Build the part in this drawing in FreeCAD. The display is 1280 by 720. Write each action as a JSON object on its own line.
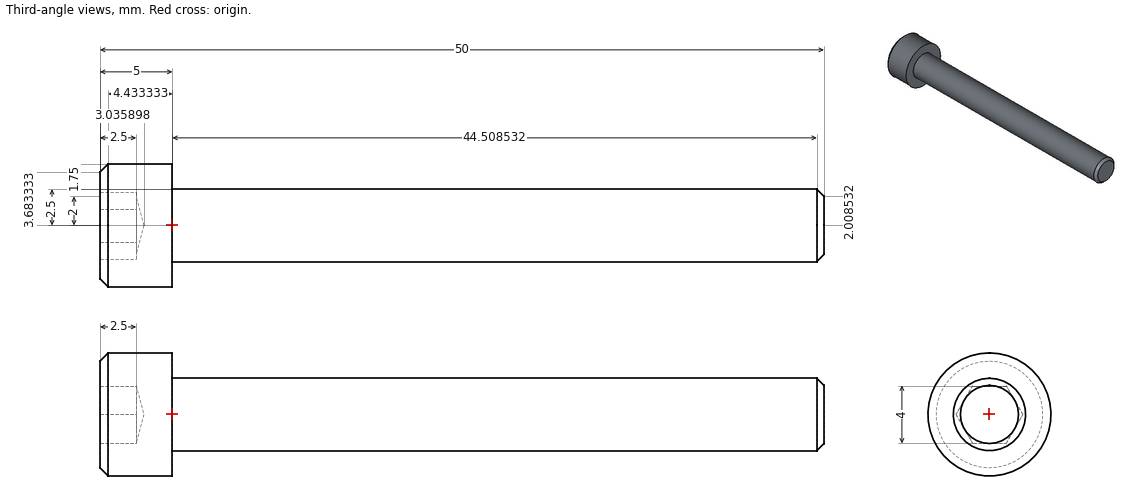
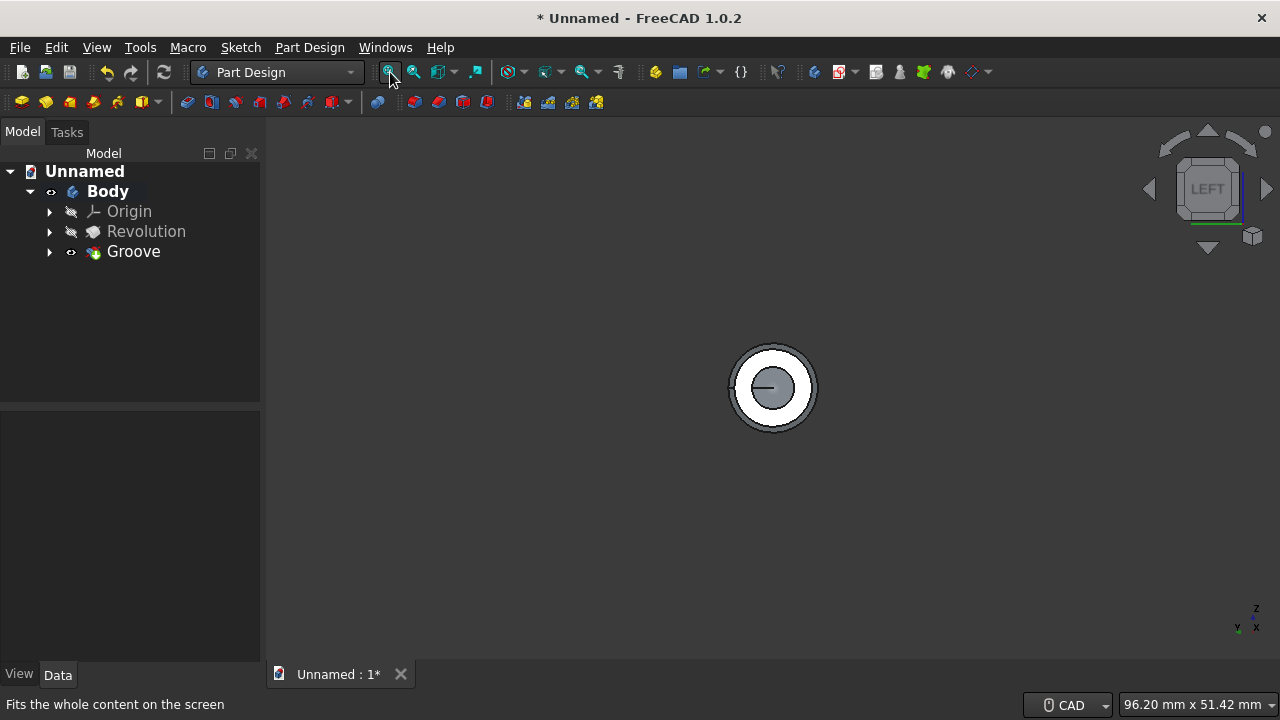
{"action": "key", "text": "2"}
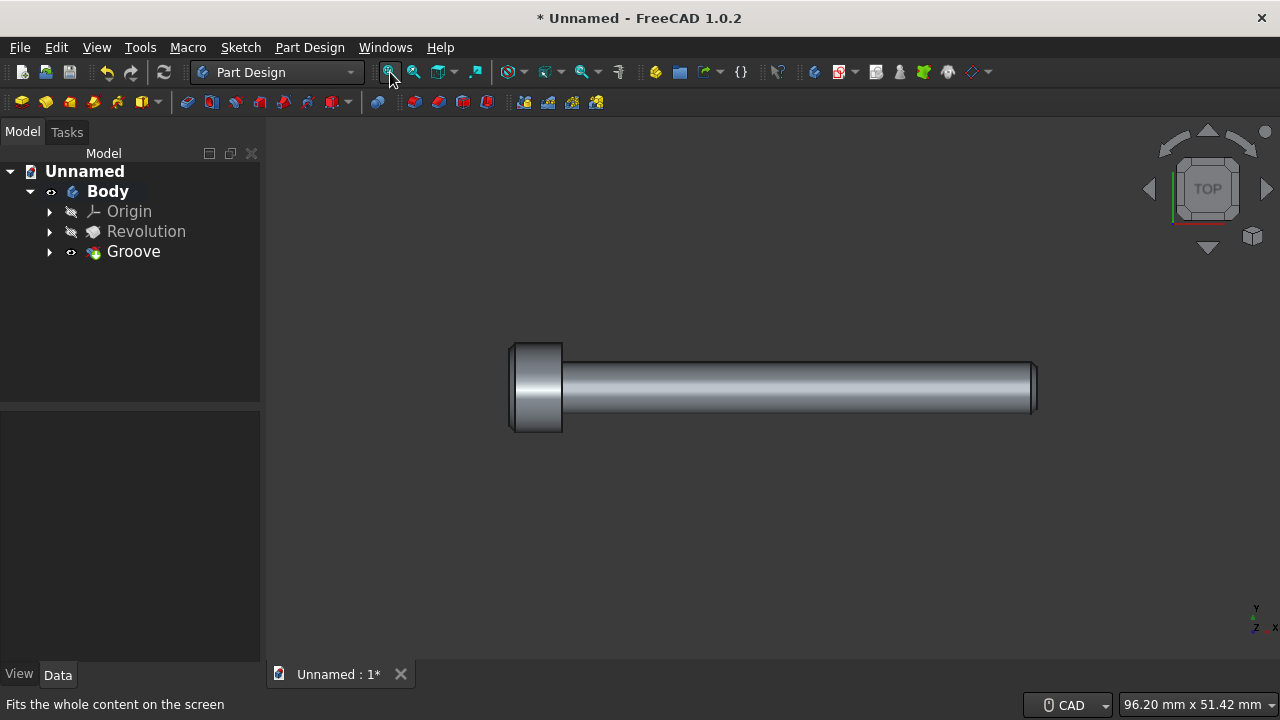
{"action": "key", "text": "1"}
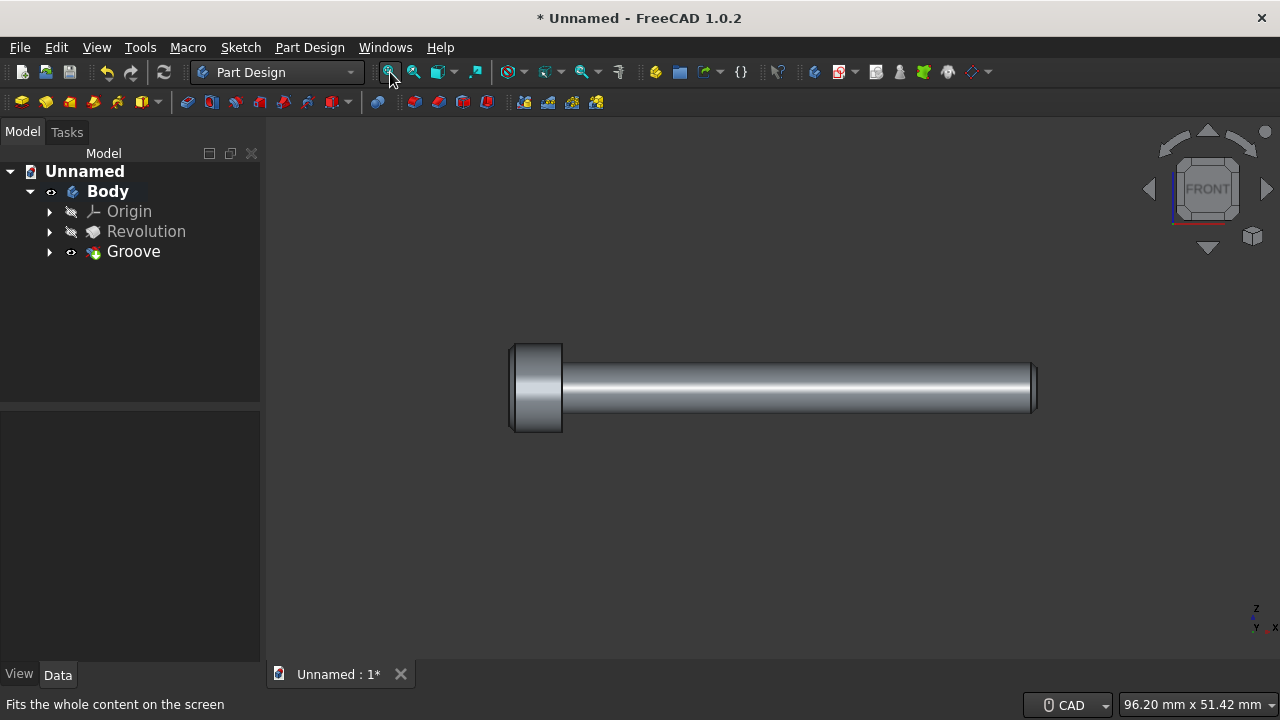
{"action": "left_click", "coordinate": [50, 212]}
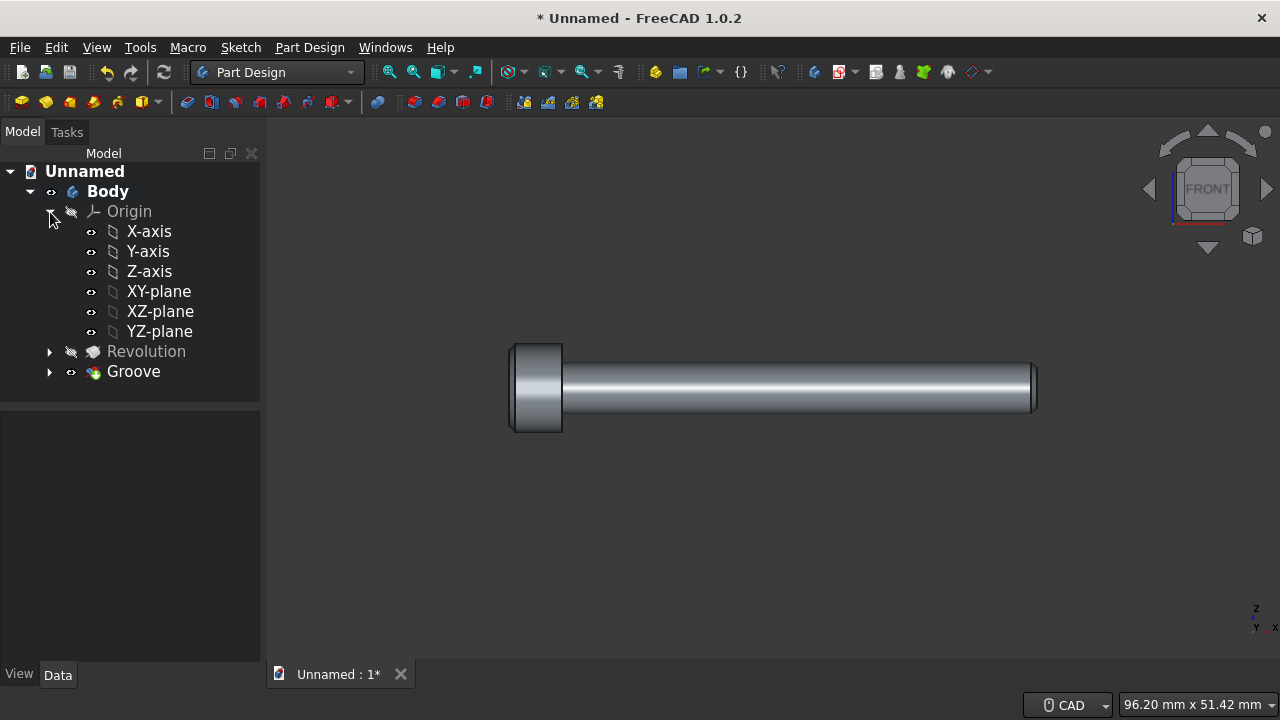
{"action": "left_click", "coordinate": [136, 332]}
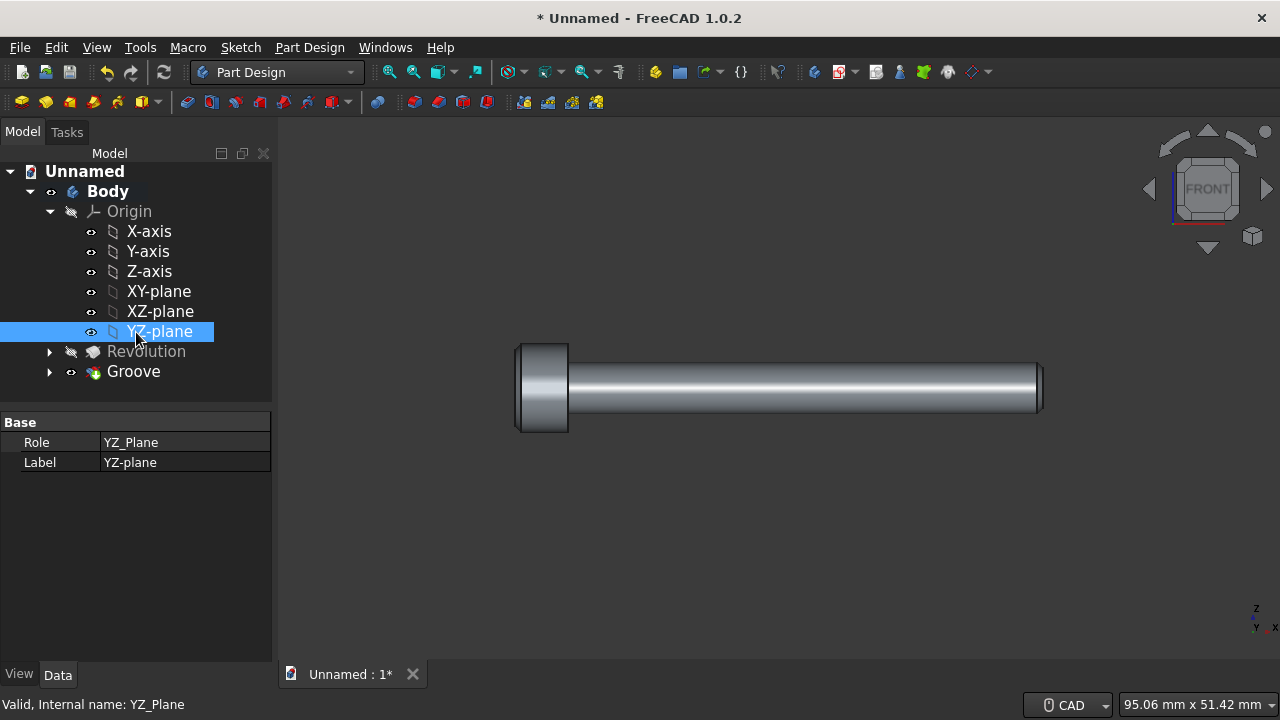
{"action": "left_click", "coordinate": [972, 72]}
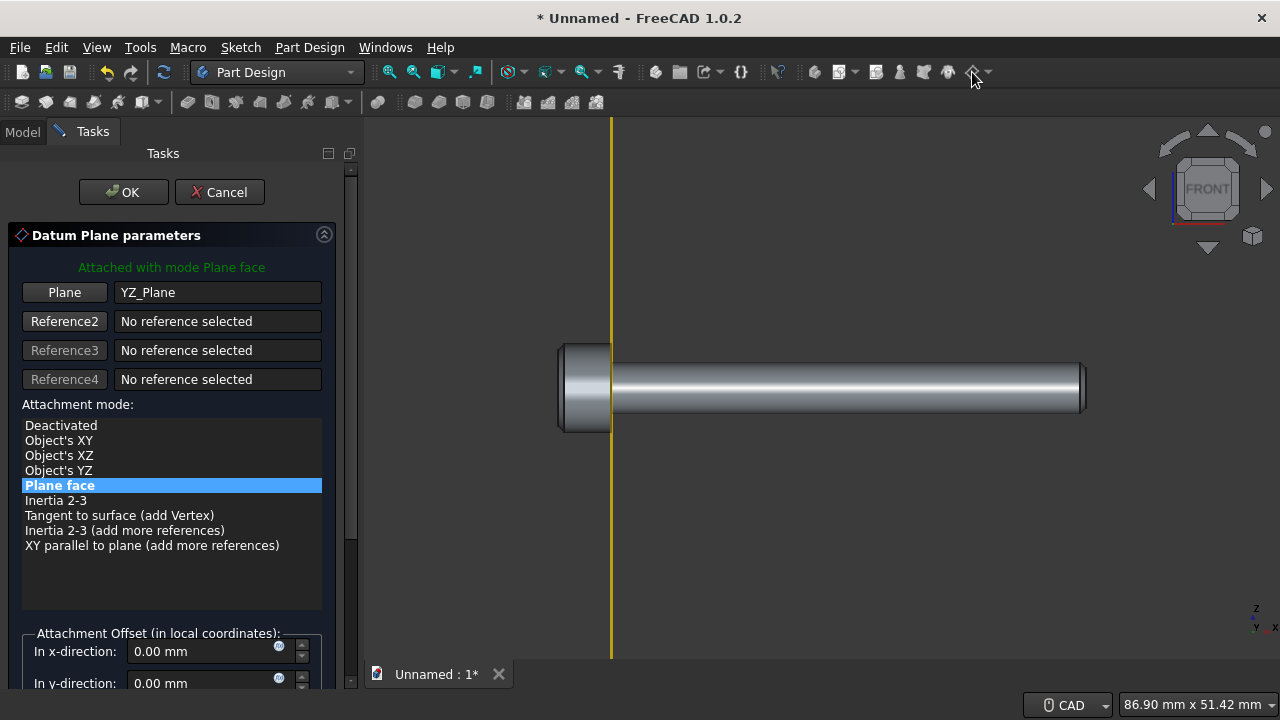
{"action": "scroll", "coordinate": [351, 426], "scroll_direction": "down", "scroll_amount": 2}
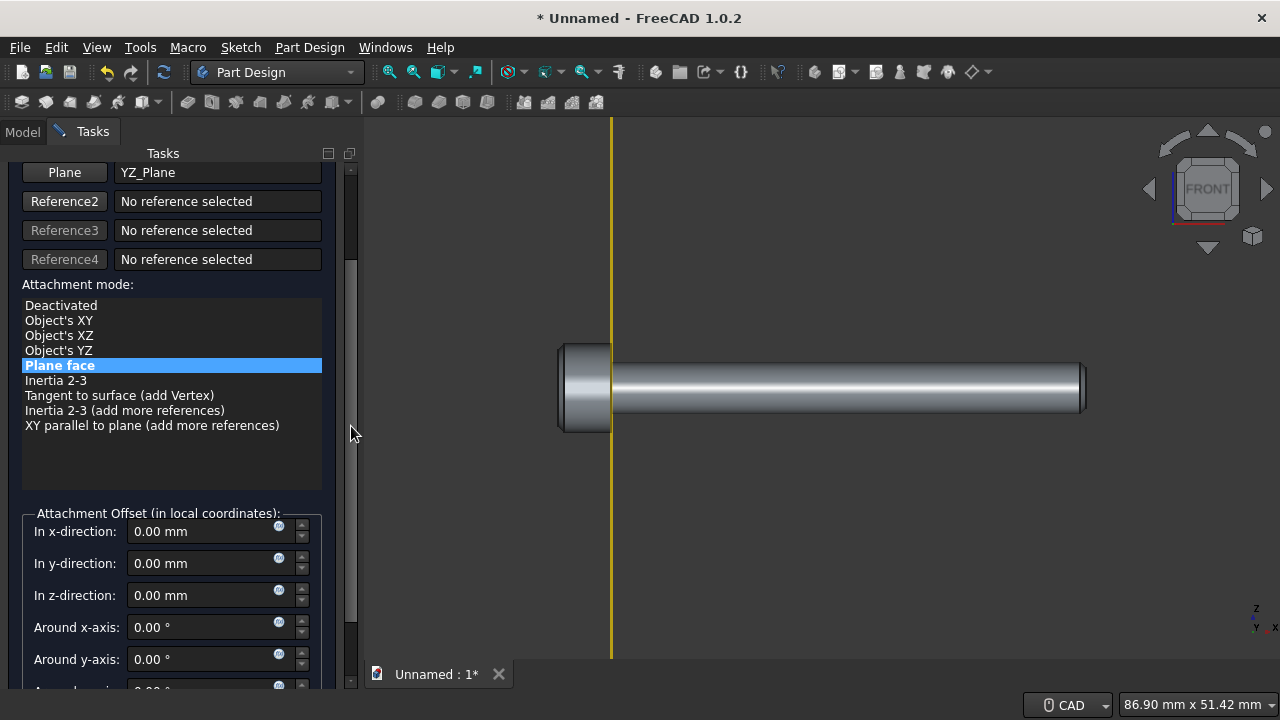
{"action": "triple_click", "coordinate": [210, 595]}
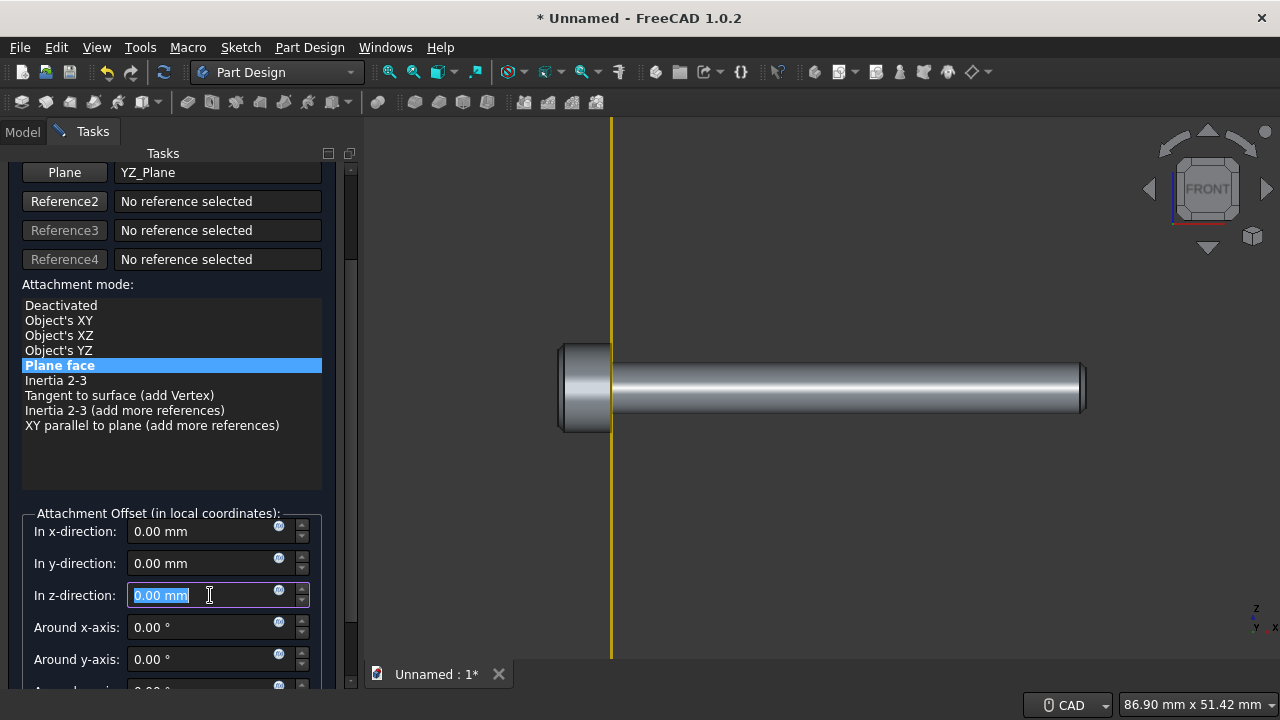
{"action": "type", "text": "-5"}
{"action": "key", "text": "Tab"}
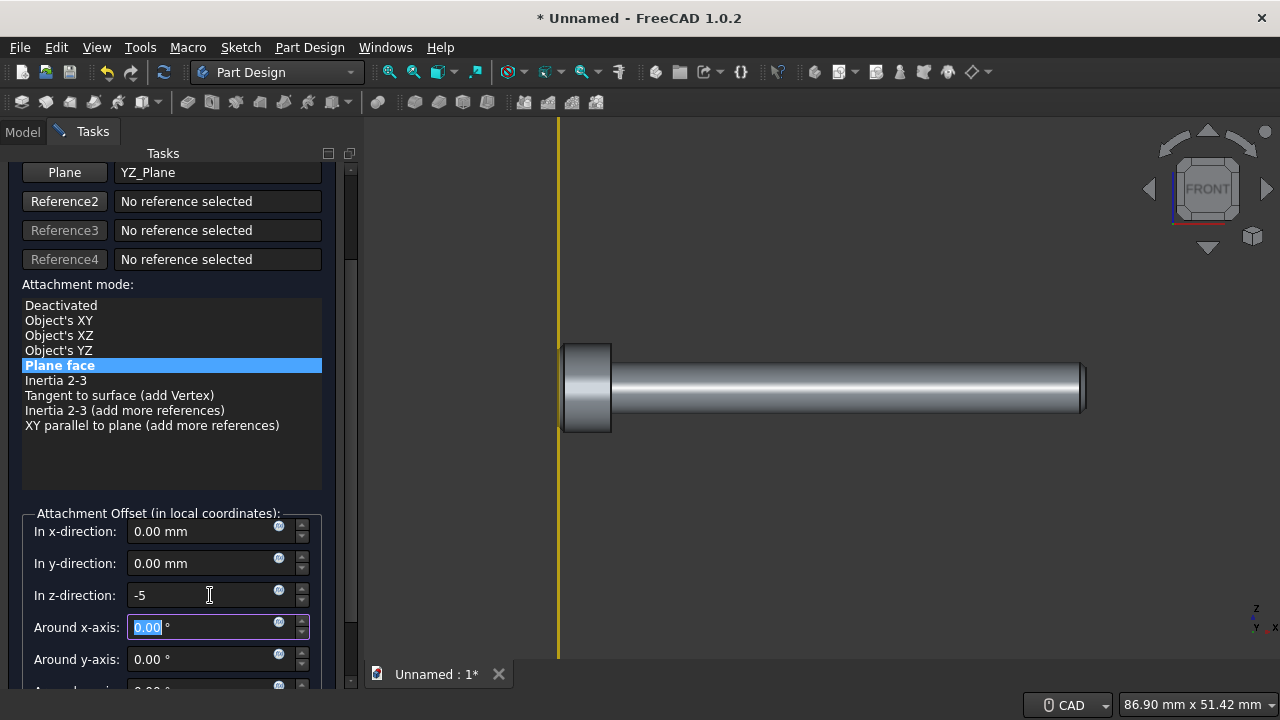
{"action": "scroll", "coordinate": [351, 426], "scroll_direction": "up", "scroll_amount": 3}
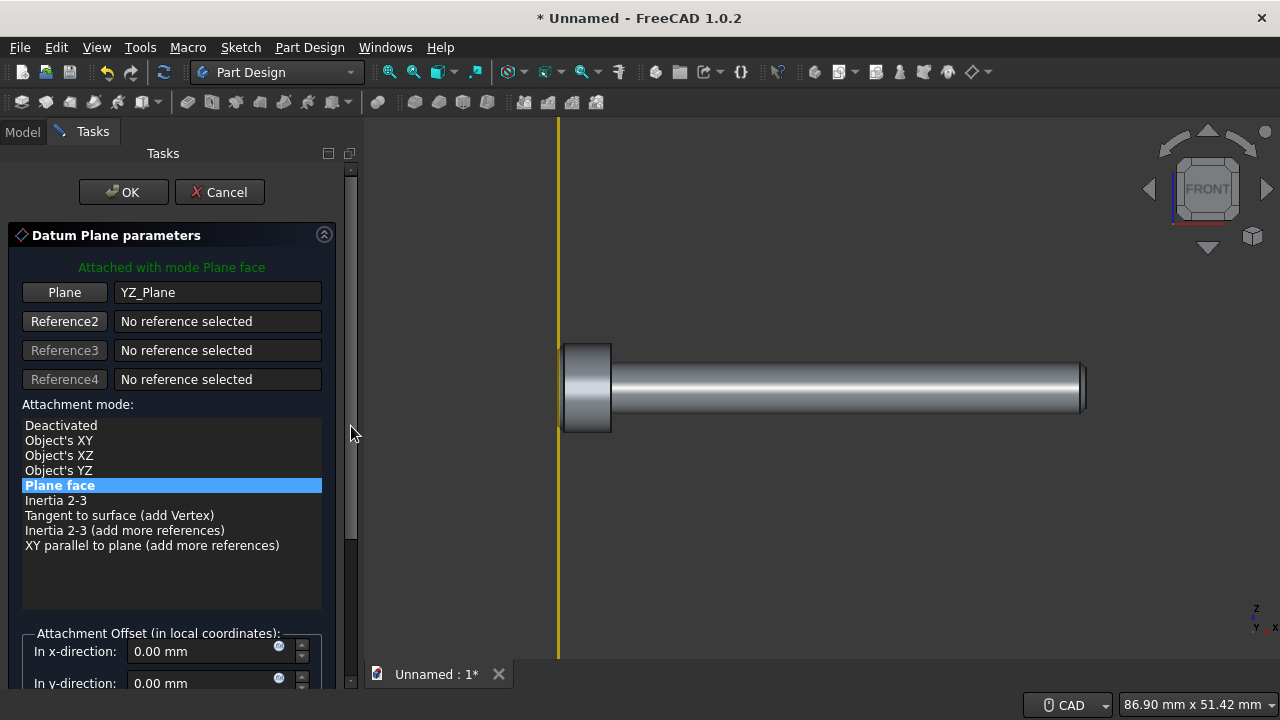
{"action": "left_click", "coordinate": [124, 192]}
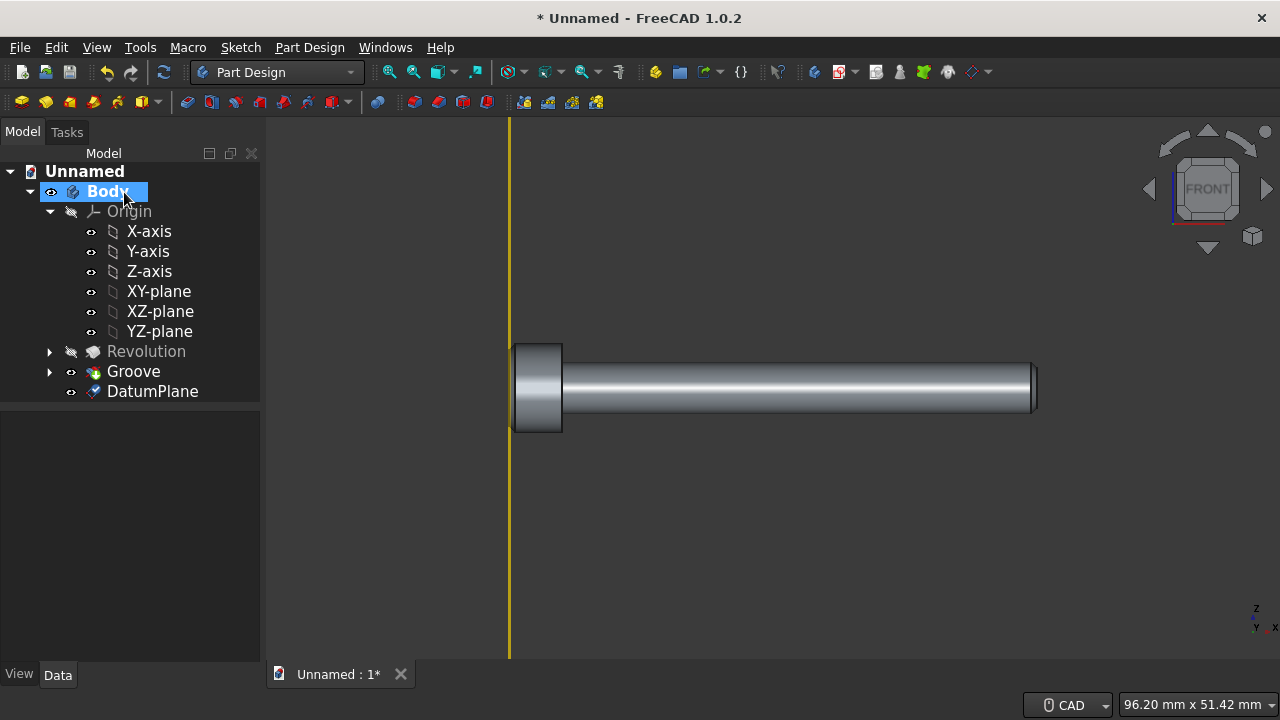
{"action": "left_click", "coordinate": [116, 392]}